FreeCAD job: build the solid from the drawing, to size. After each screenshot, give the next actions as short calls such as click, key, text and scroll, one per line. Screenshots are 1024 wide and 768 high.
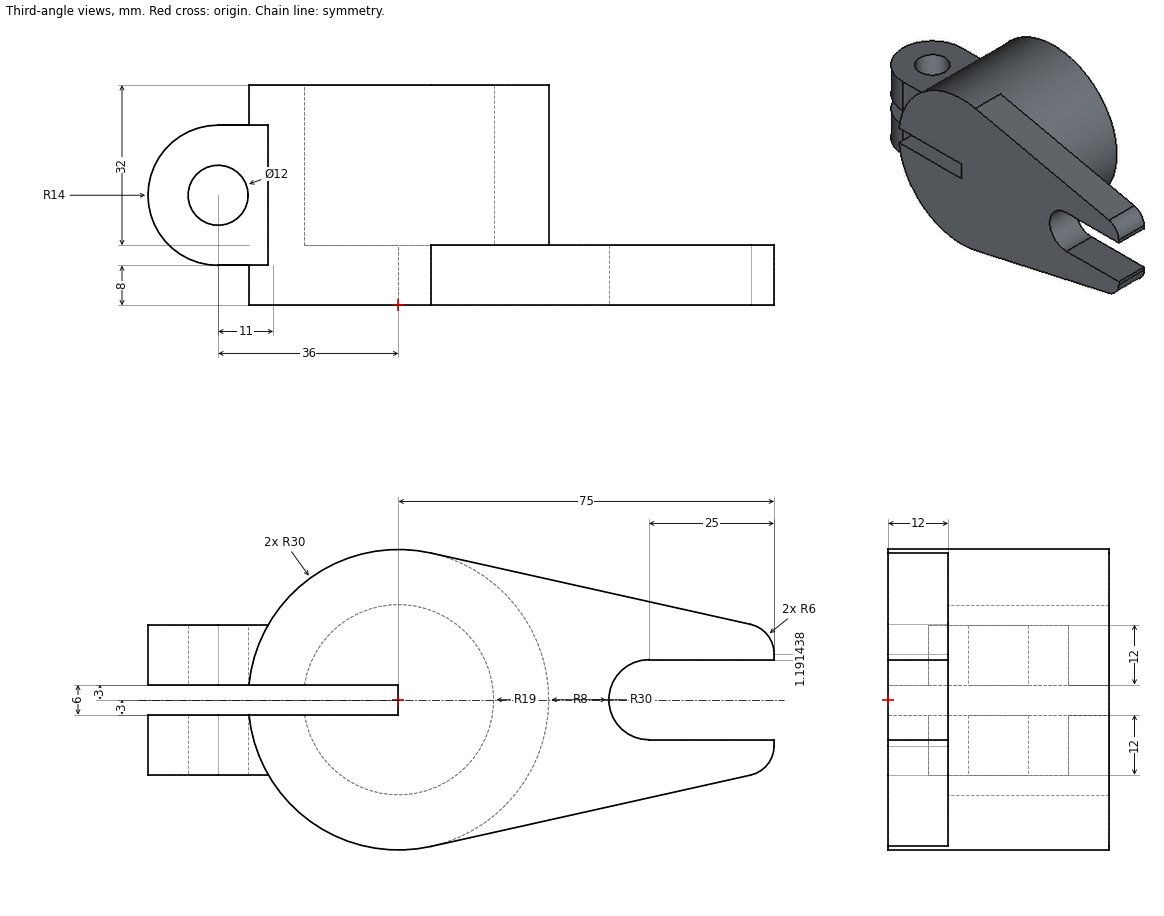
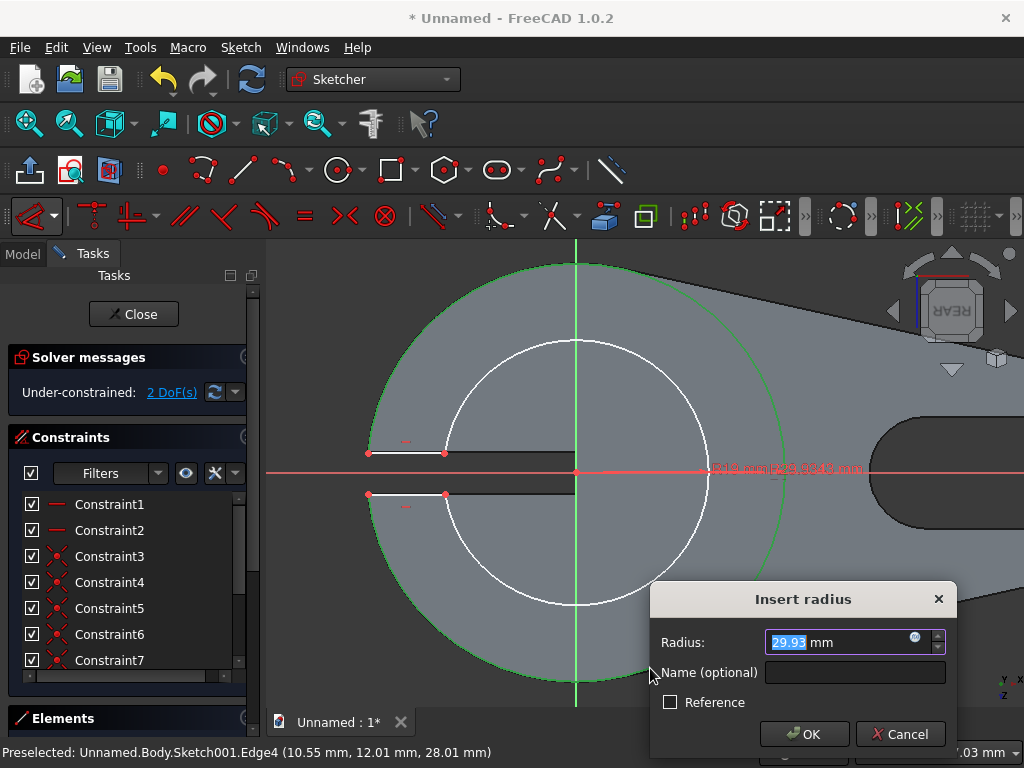
text(30)
key(Return)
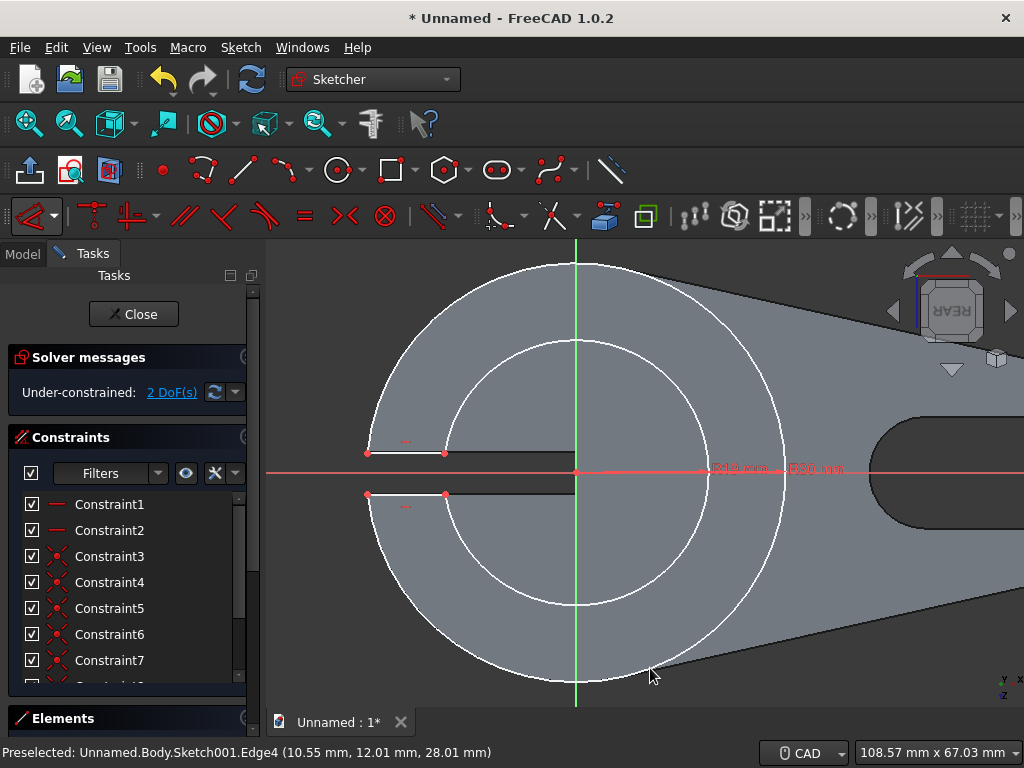
scroll(368, 453, up, 4)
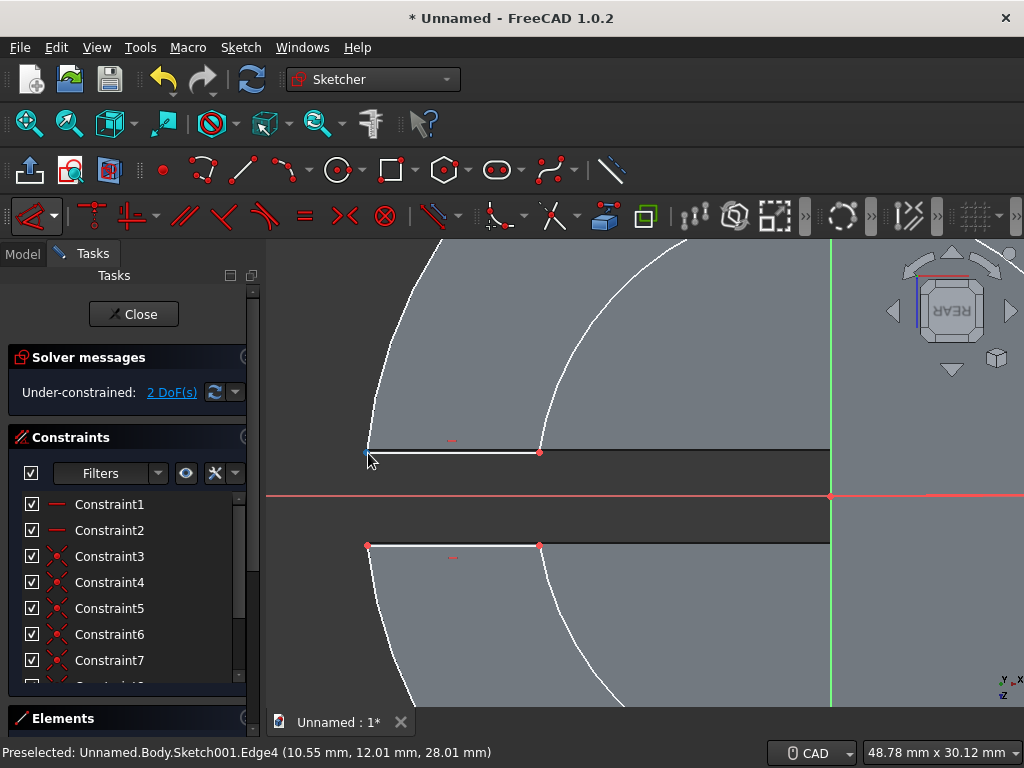
click(367, 453)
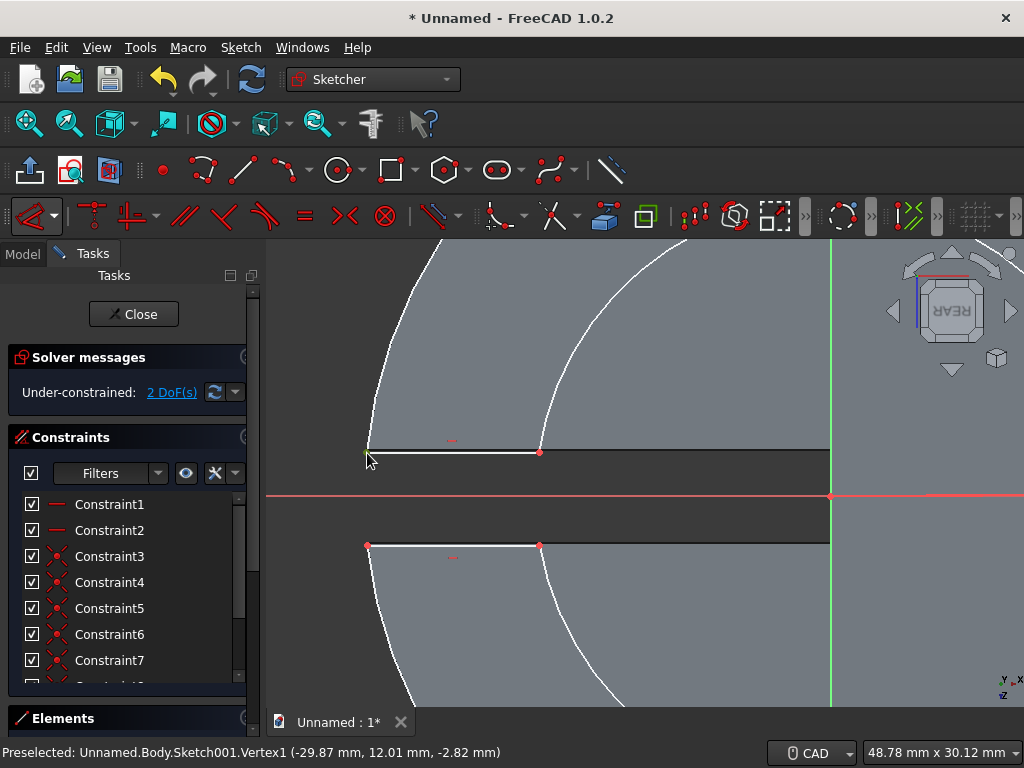
key(i)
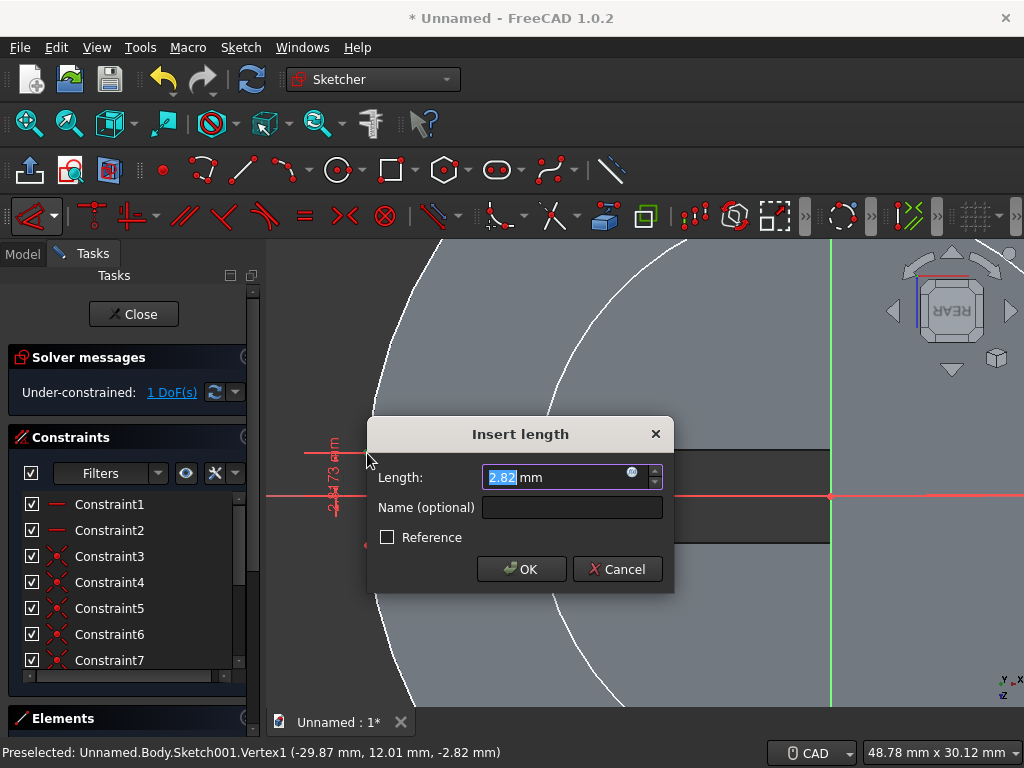
text(3)
key(Return)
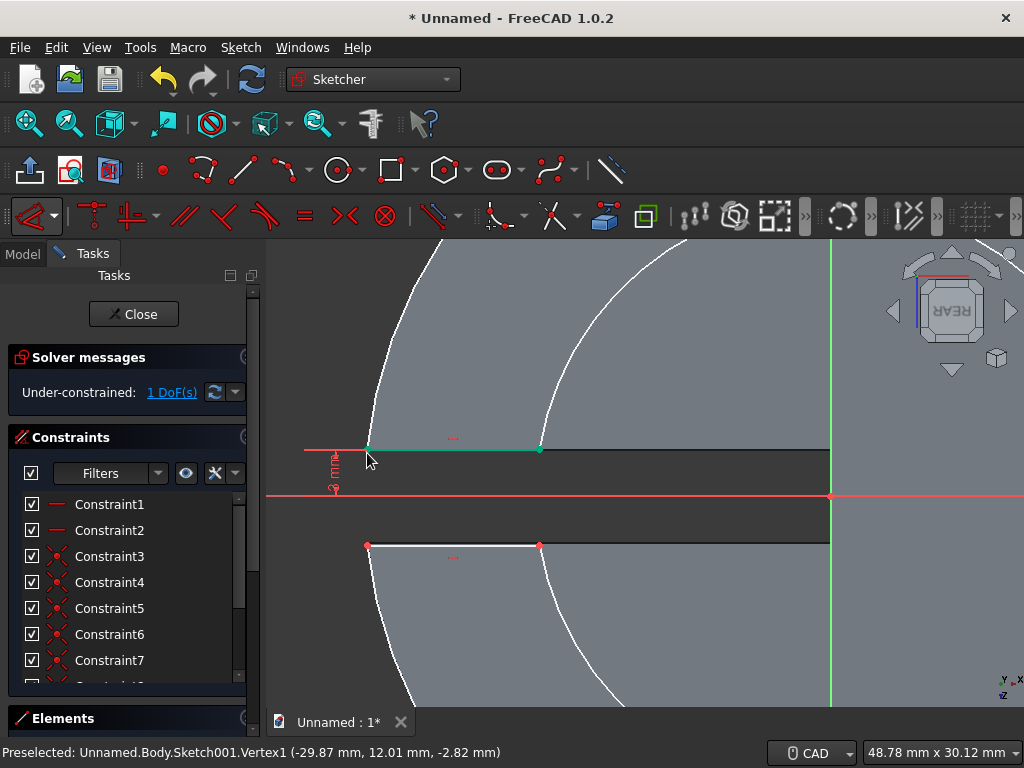
click(540, 546)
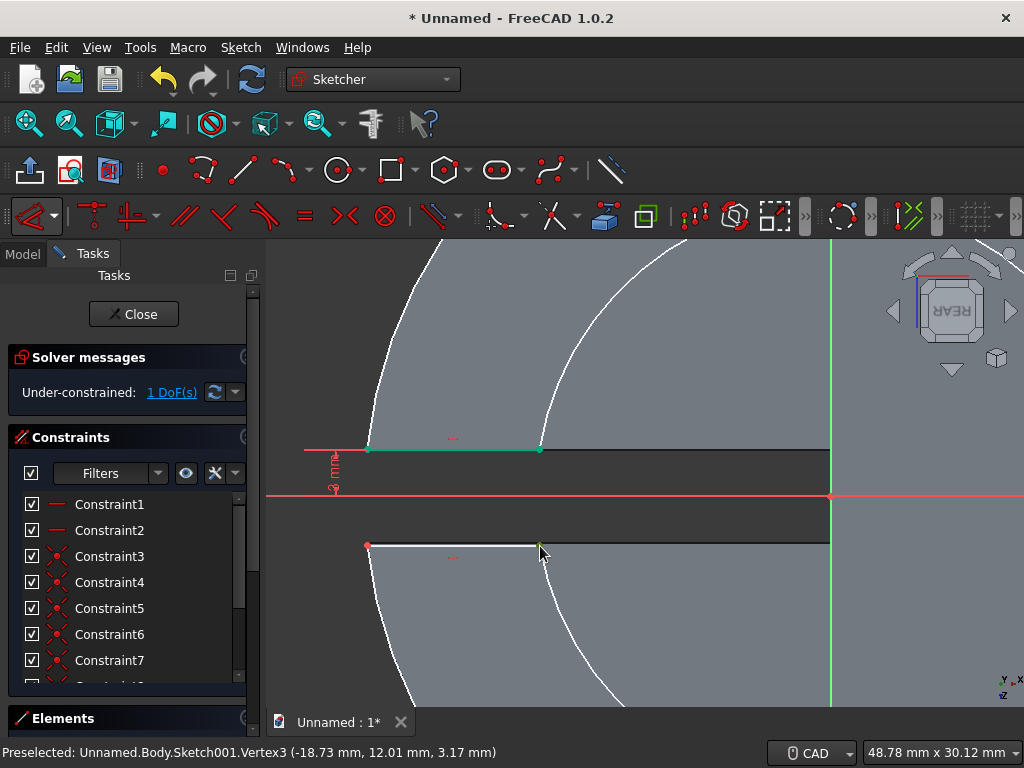
key(i)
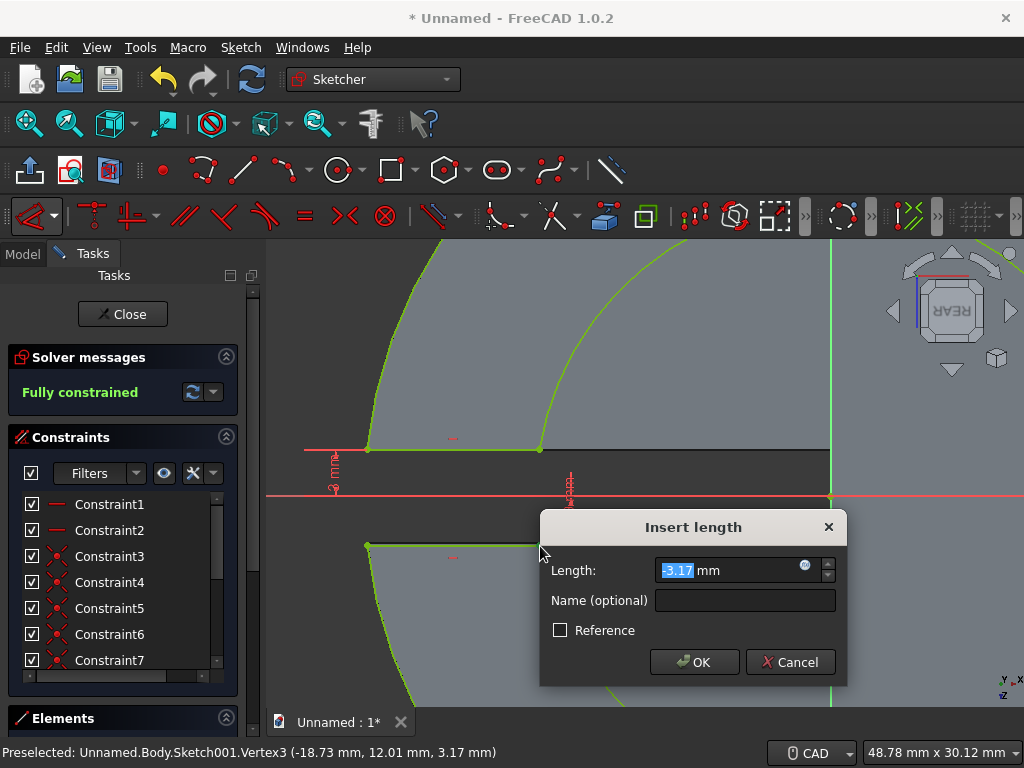
text(-3)
key(Return)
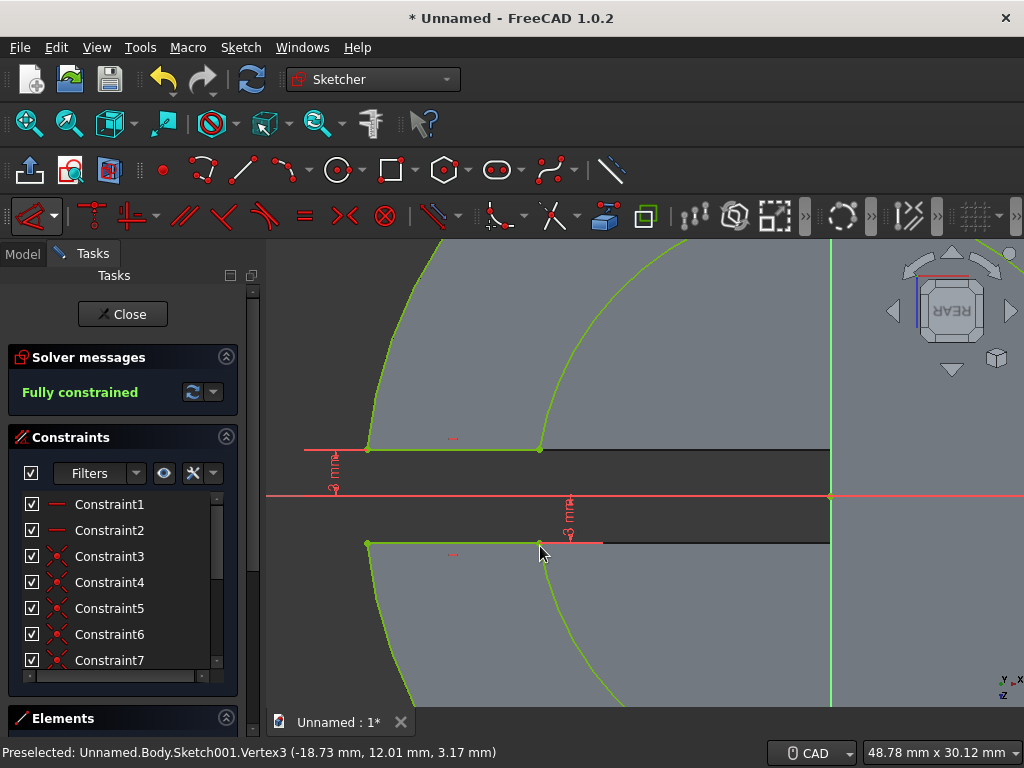
click(123, 314)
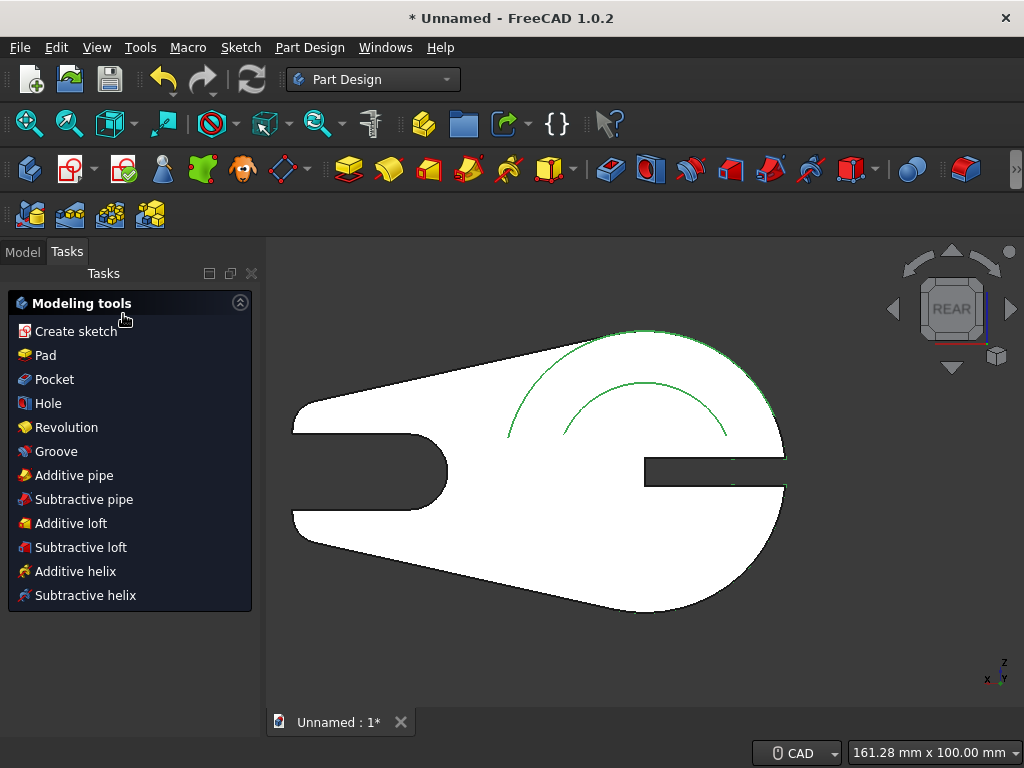
click(350, 170)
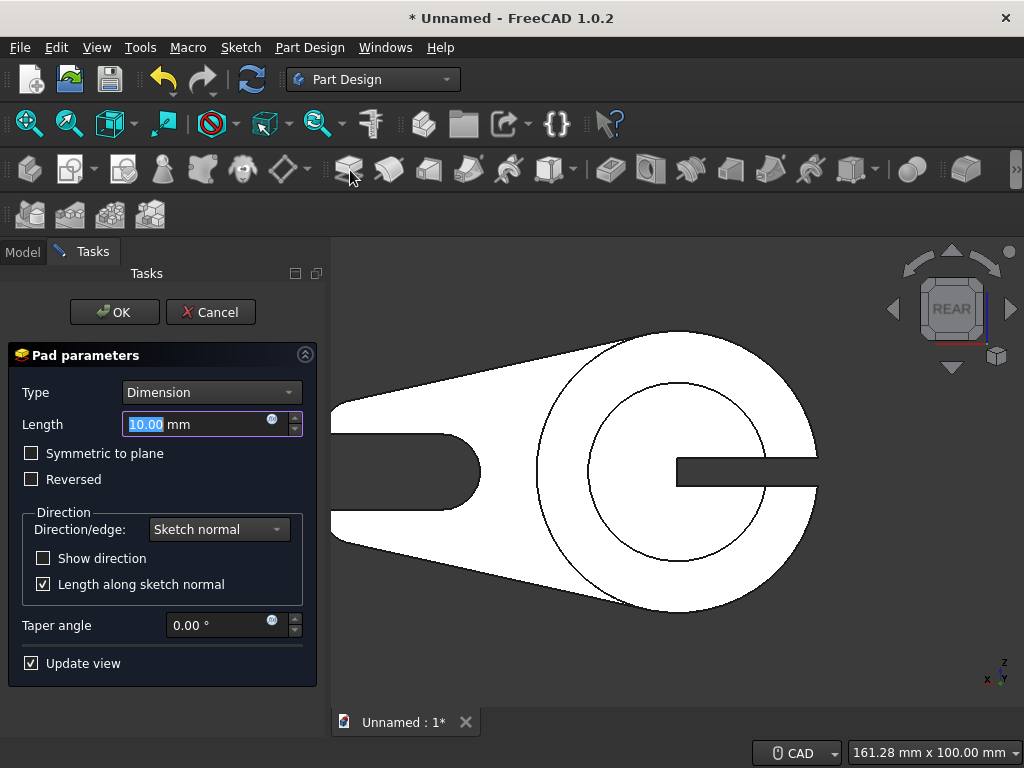
text(32)
key(Tab)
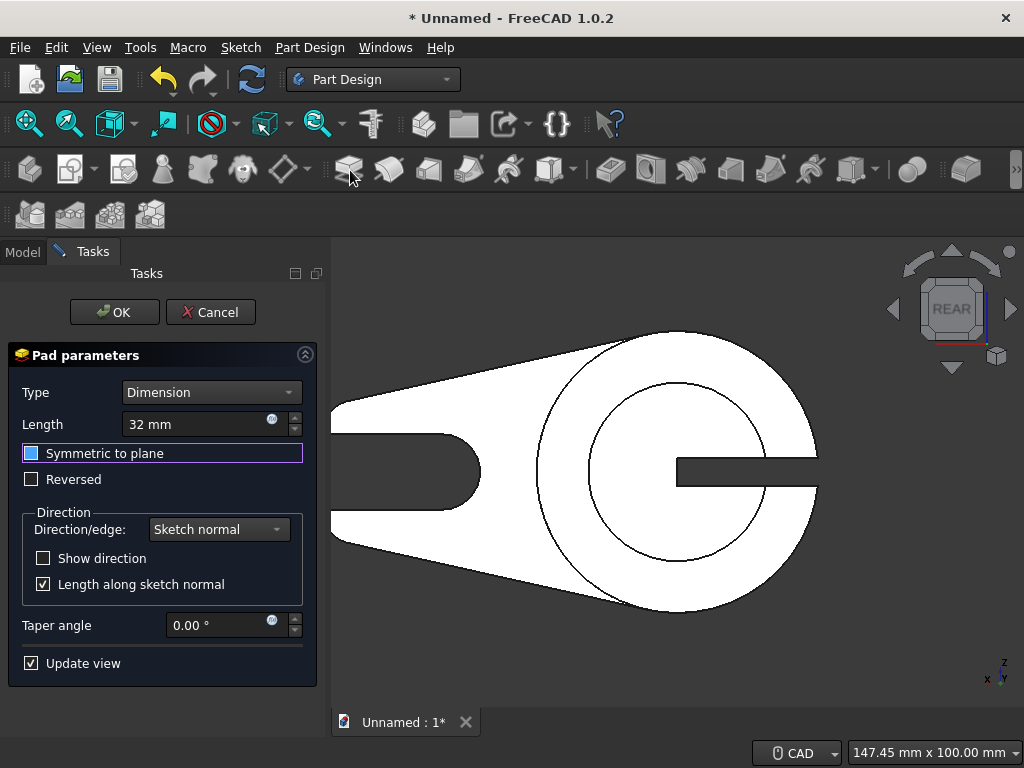
click(115, 312)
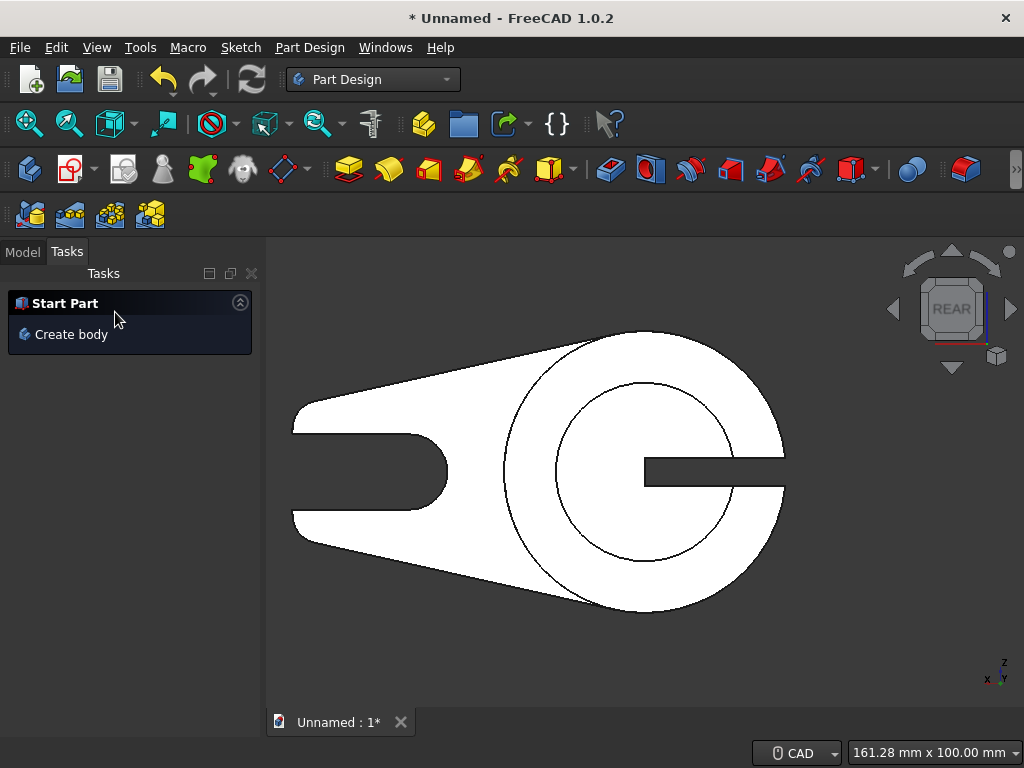
click(23, 251)